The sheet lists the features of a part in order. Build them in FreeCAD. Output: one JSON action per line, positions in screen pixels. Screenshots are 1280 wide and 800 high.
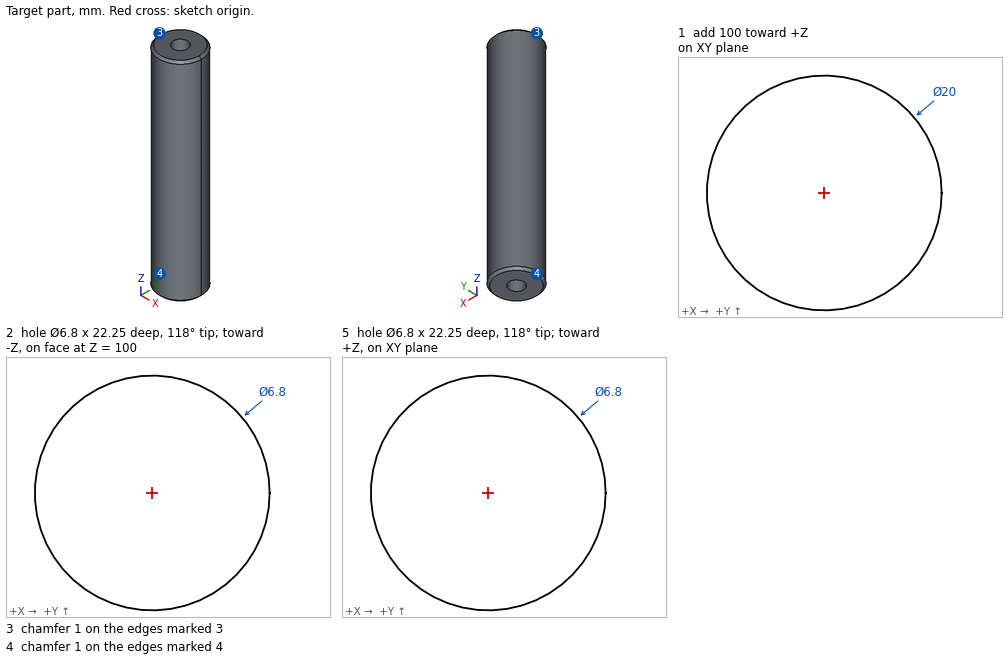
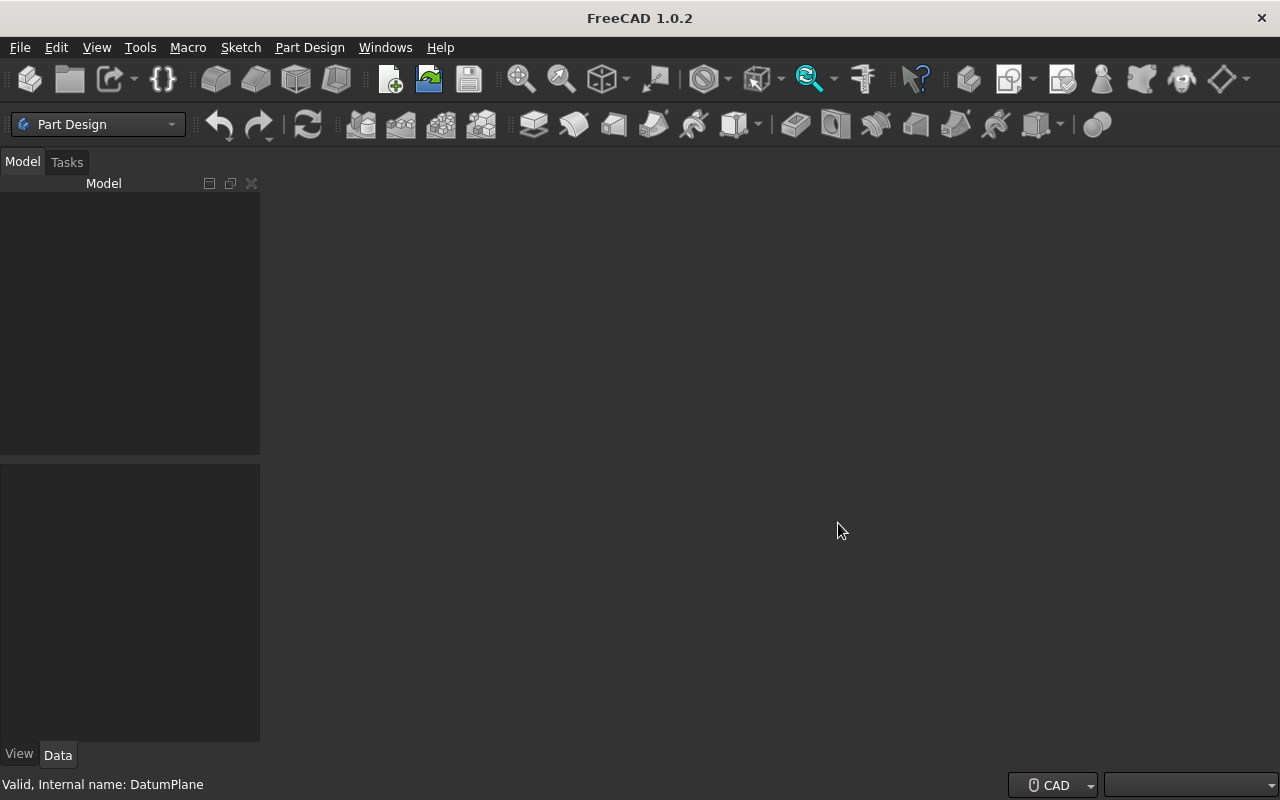
{"action": "key", "text": "ctrl+n"}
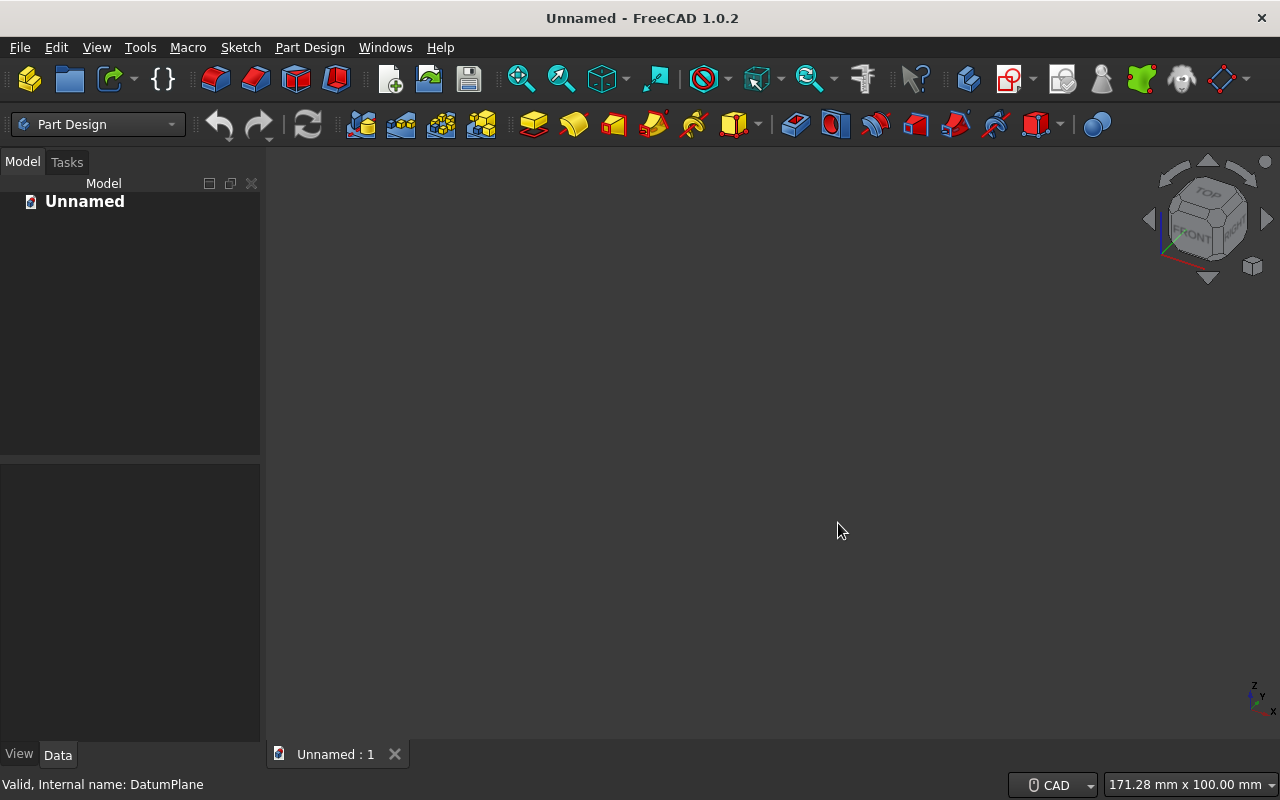
{"action": "left_click", "coordinate": [1010, 80]}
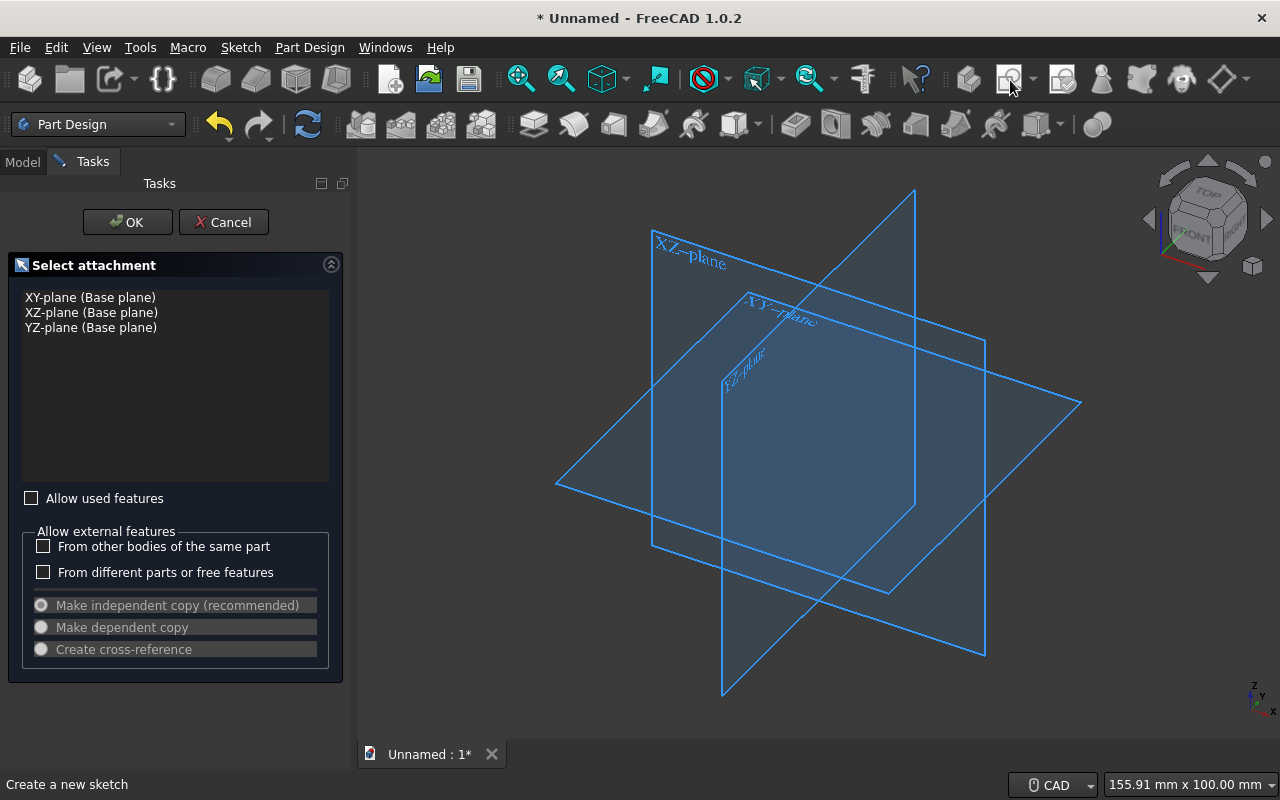
{"action": "left_click", "coordinate": [82, 298]}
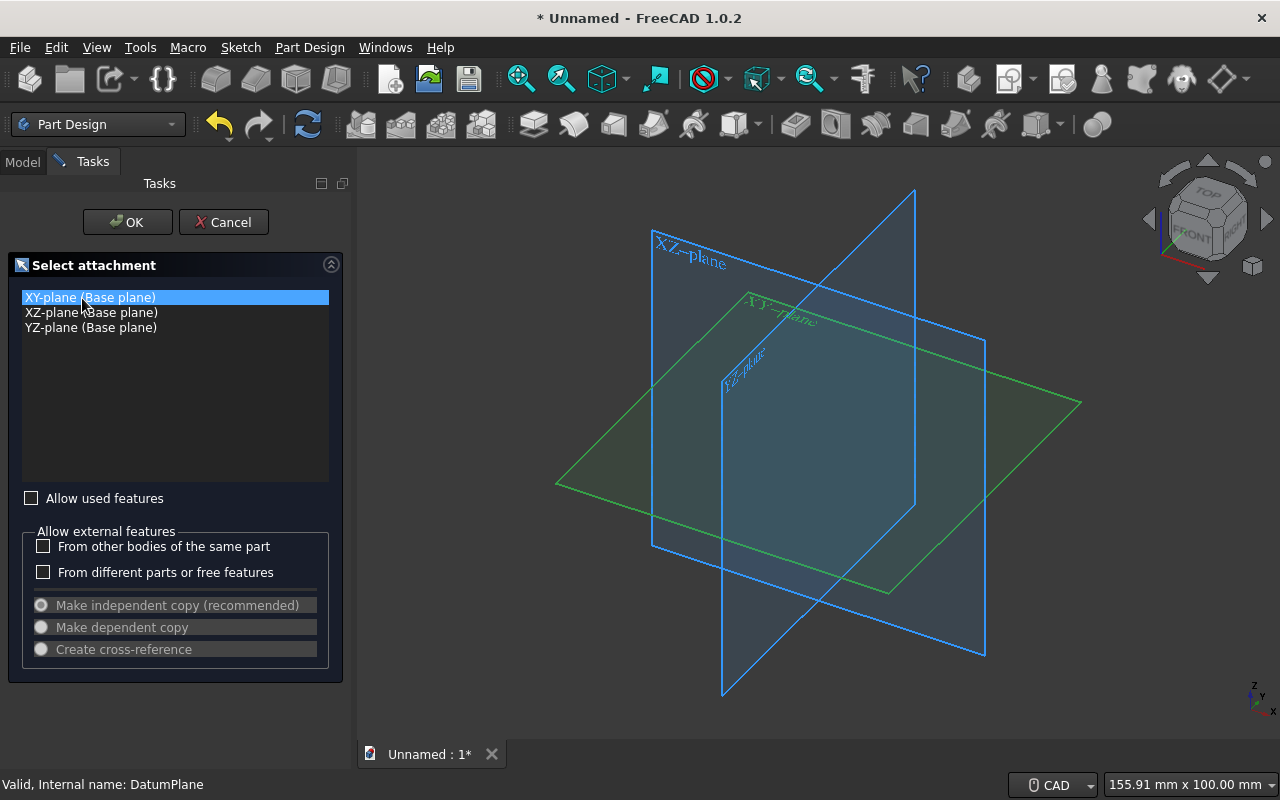
{"action": "left_click", "coordinate": [128, 222]}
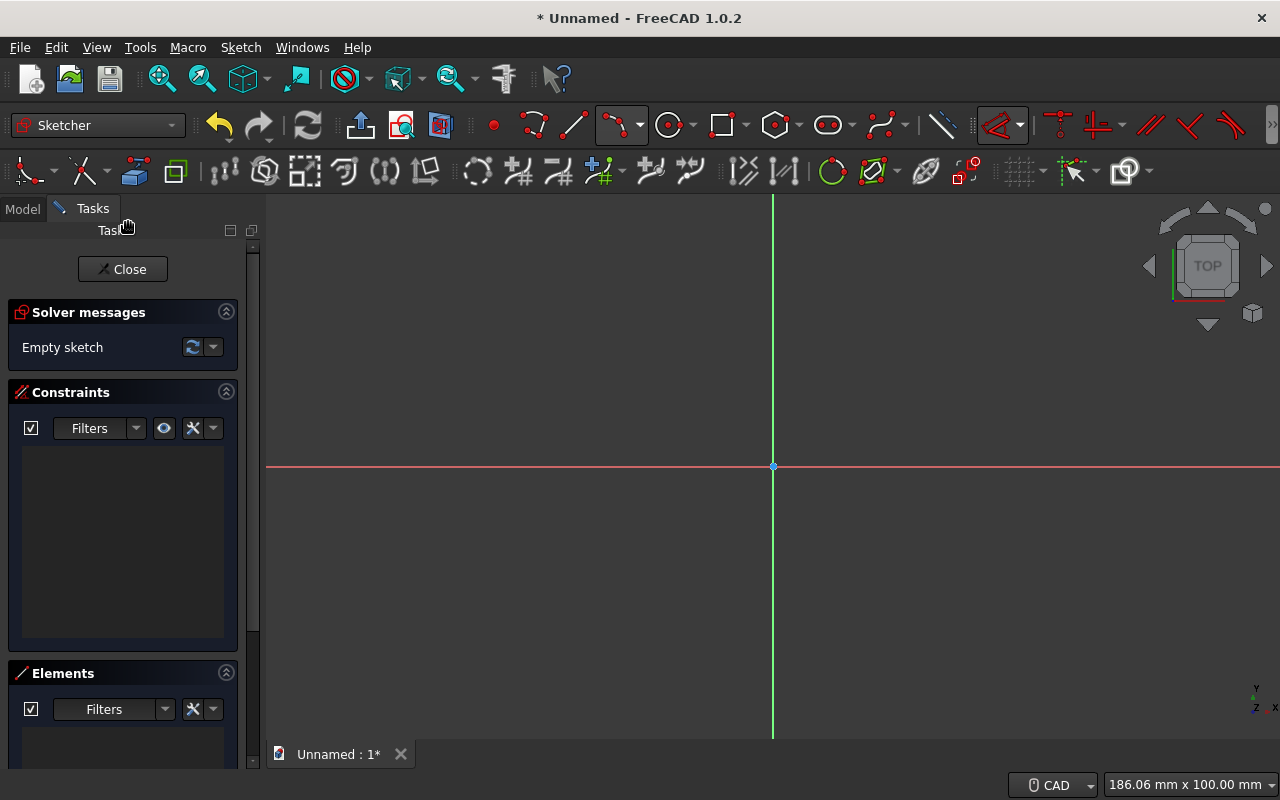
{"action": "scroll", "coordinate": [803, 466], "scroll_direction": "up", "scroll_amount": 6}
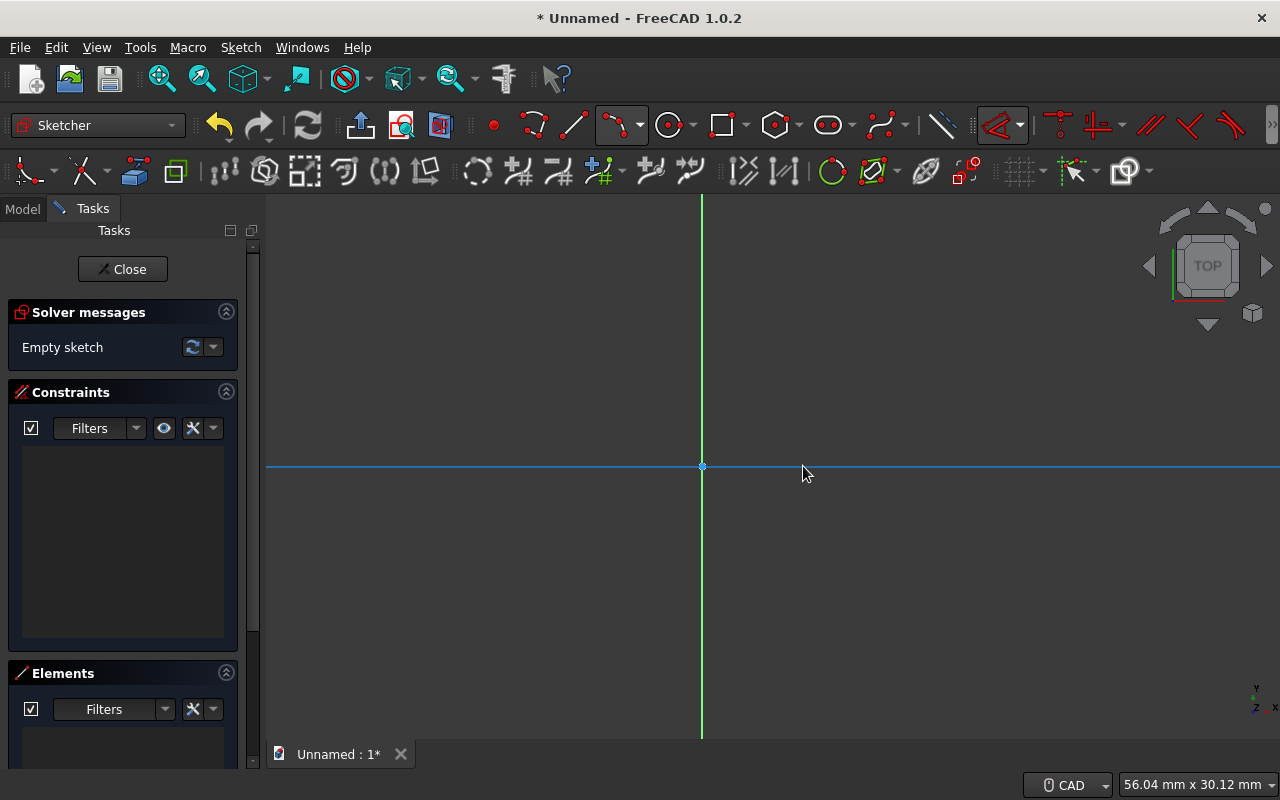
{"action": "left_click", "coordinate": [670, 126]}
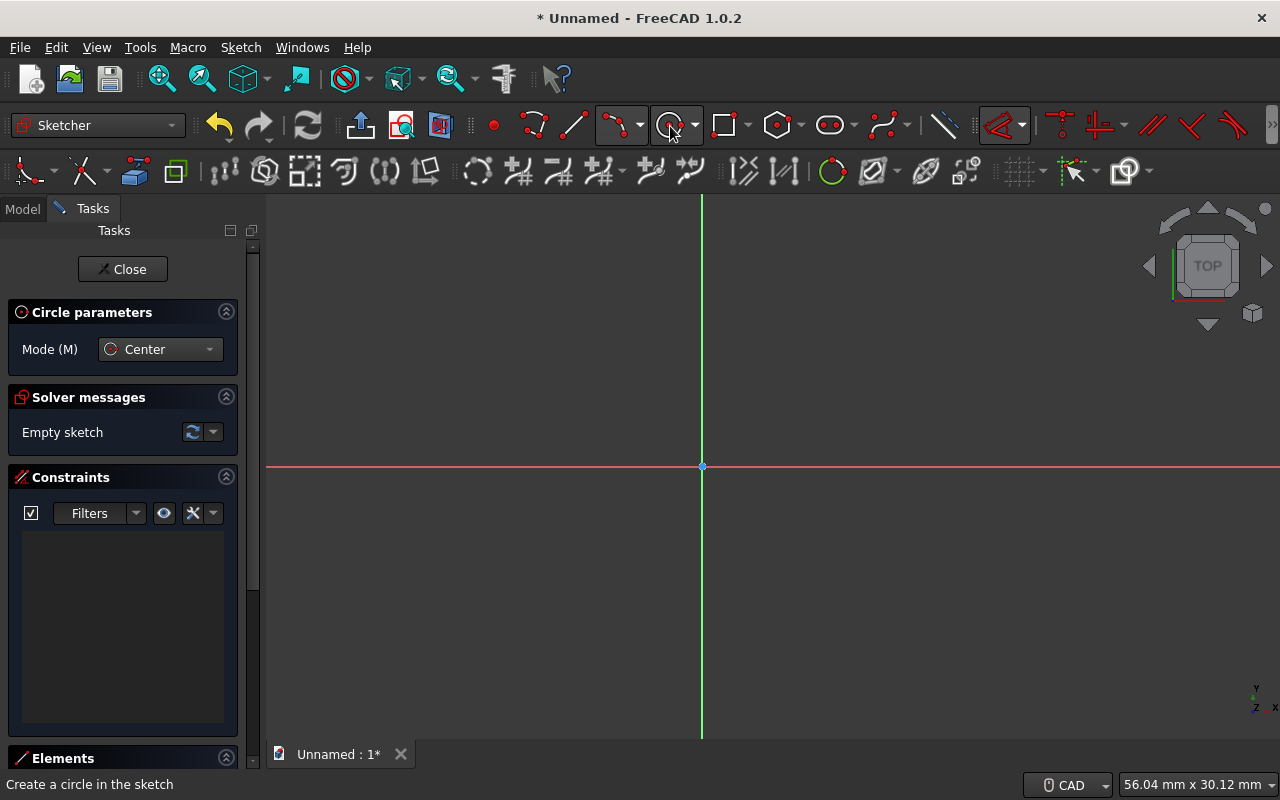
{"action": "left_click", "coordinate": [702, 466]}
{"action": "mouse_move", "coordinate": [830, 339]}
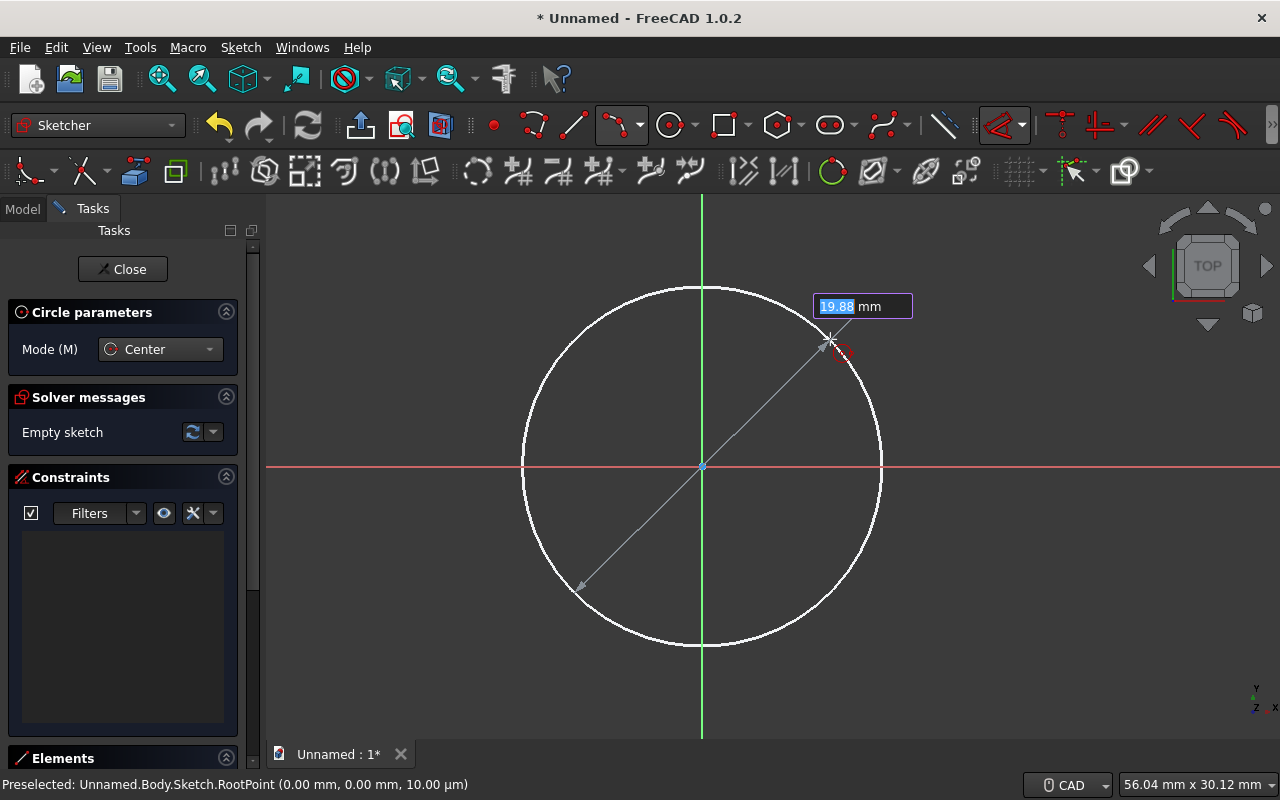
{"action": "type", "text": "20"}
{"action": "key", "text": "Return"}
{"action": "key", "text": "Escape"}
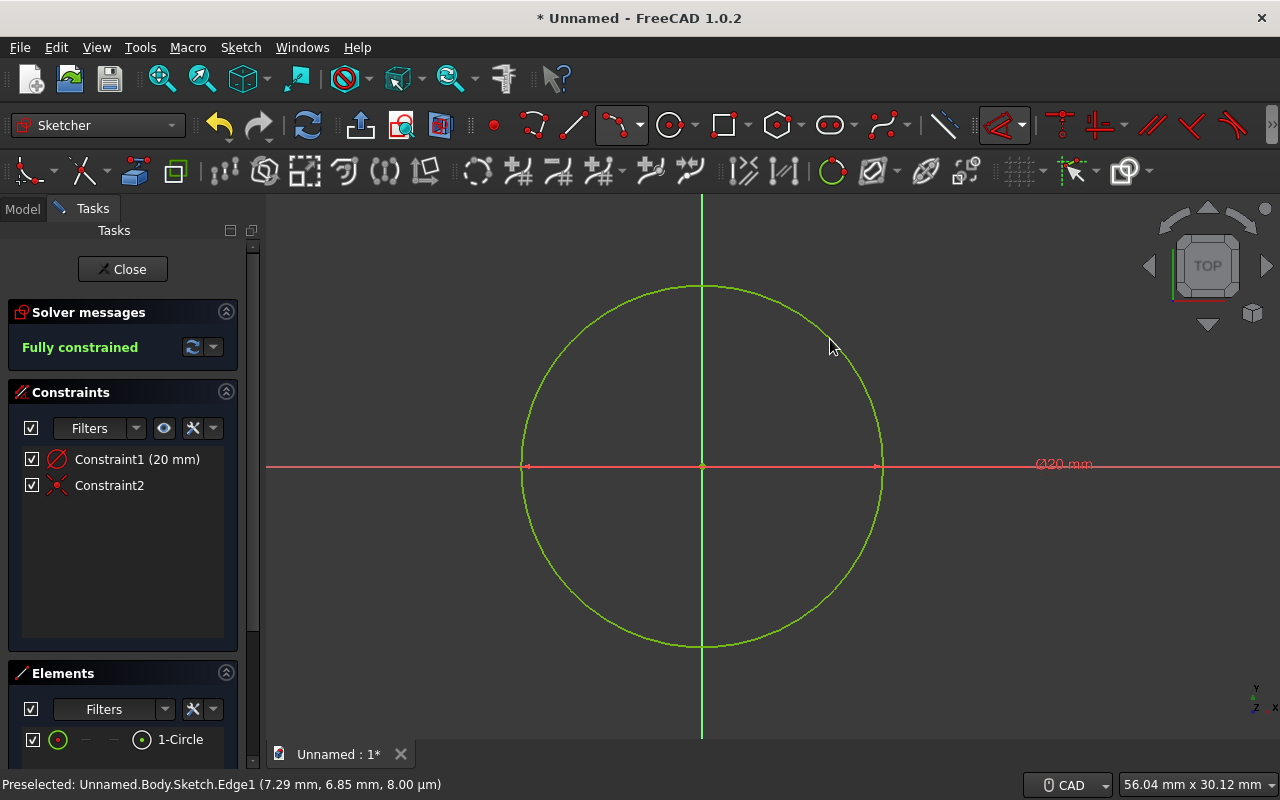
{"action": "left_click", "coordinate": [123, 269]}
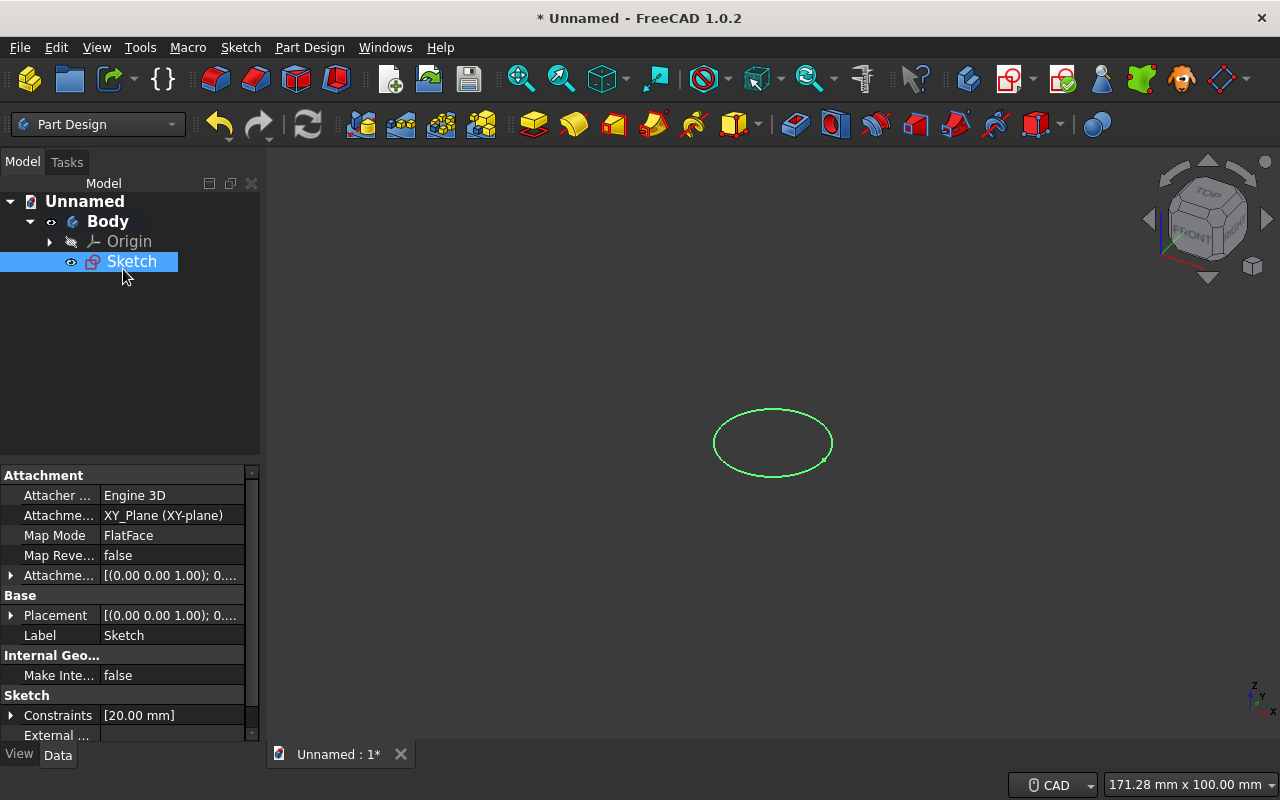
{"action": "left_click", "coordinate": [534, 124]}